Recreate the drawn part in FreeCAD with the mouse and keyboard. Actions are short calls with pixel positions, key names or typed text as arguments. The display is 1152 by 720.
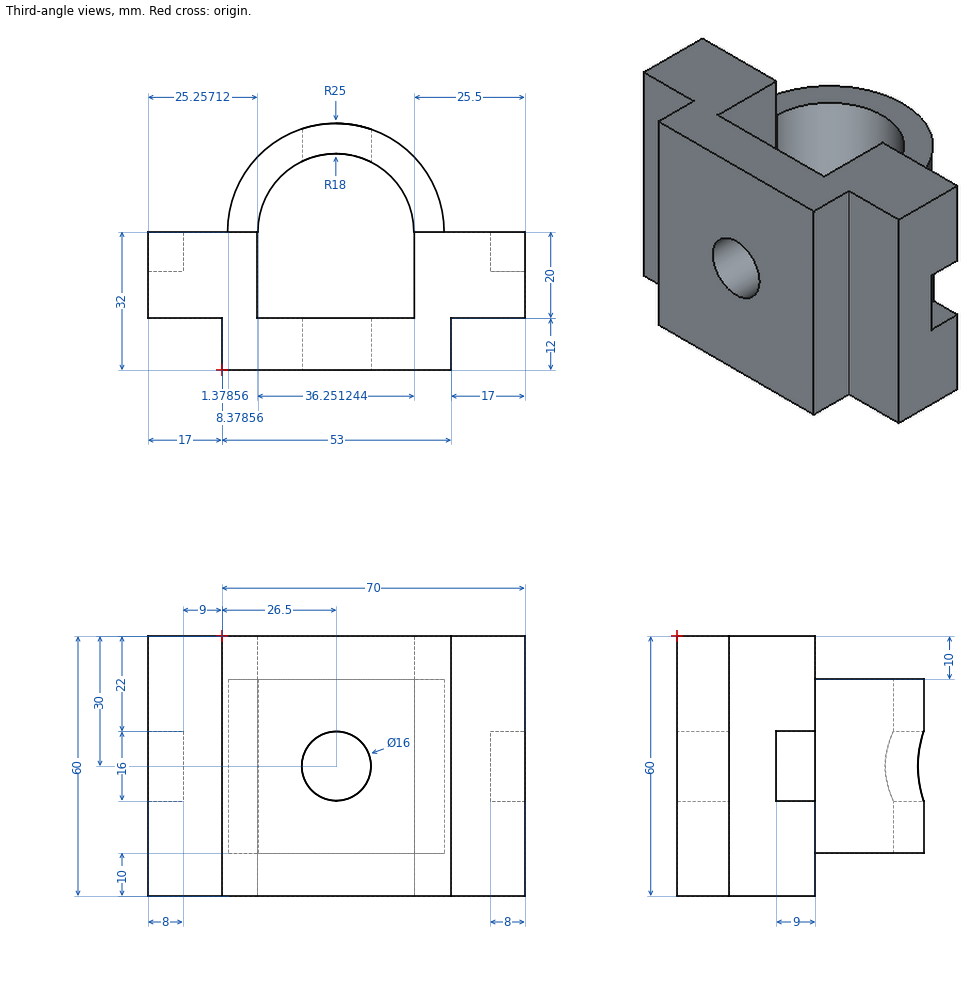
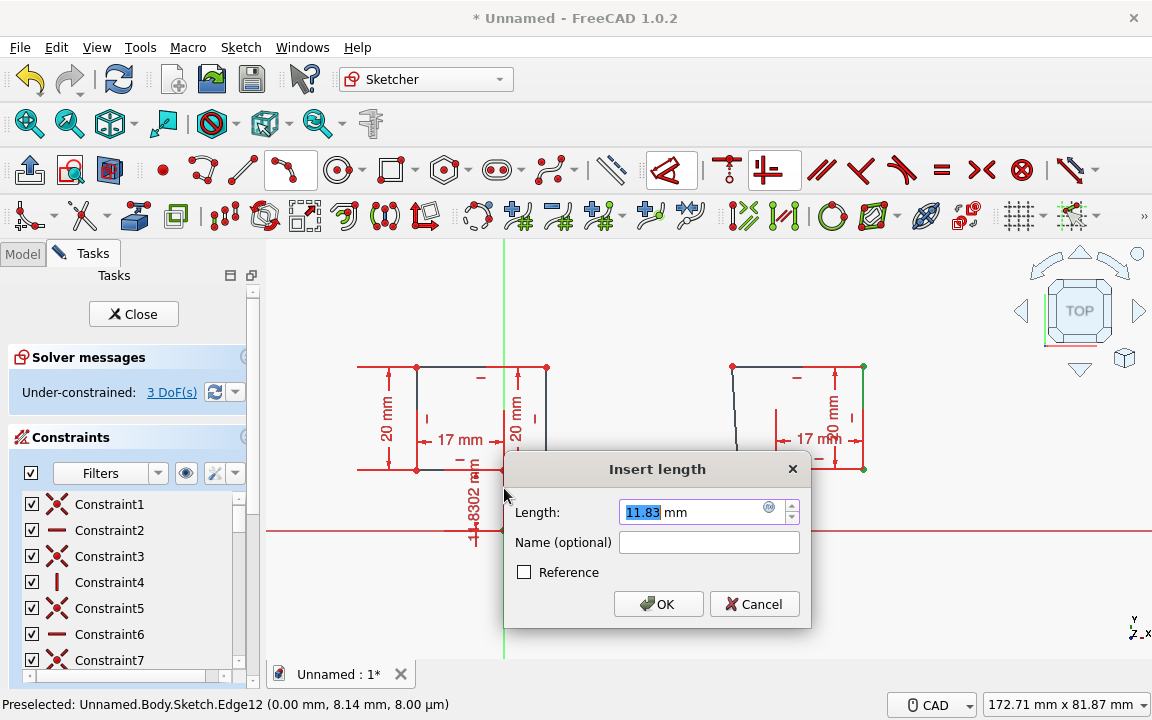
text(12)
key(Return)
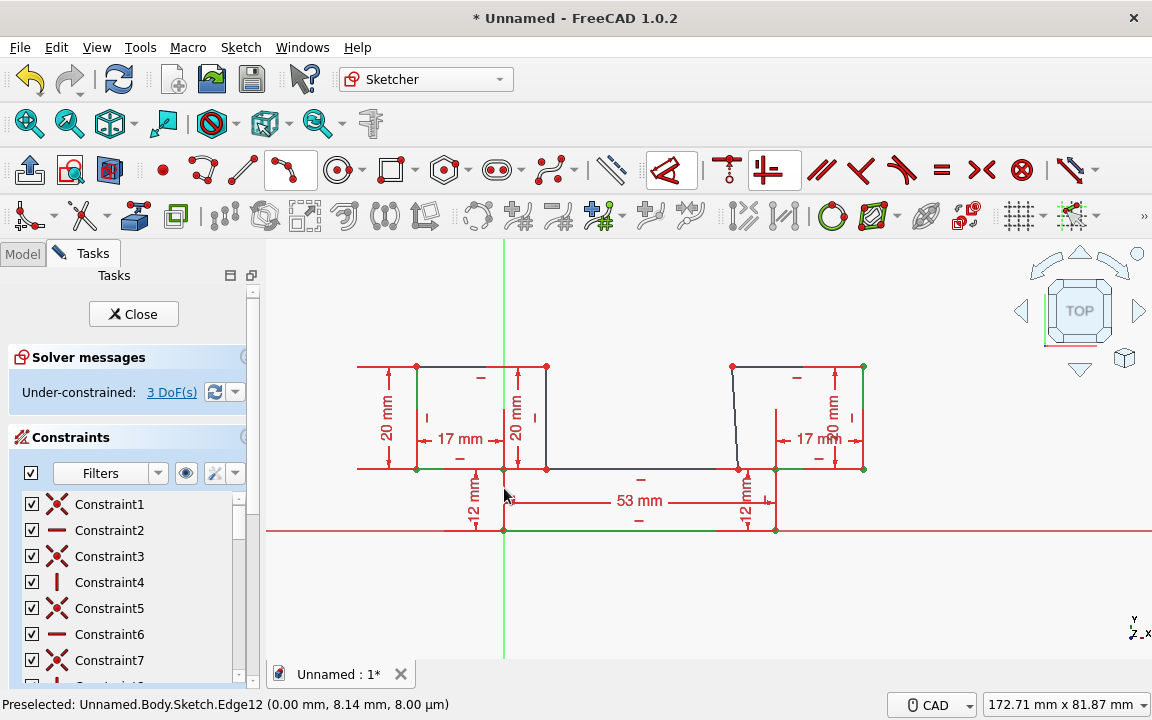
click(824, 367)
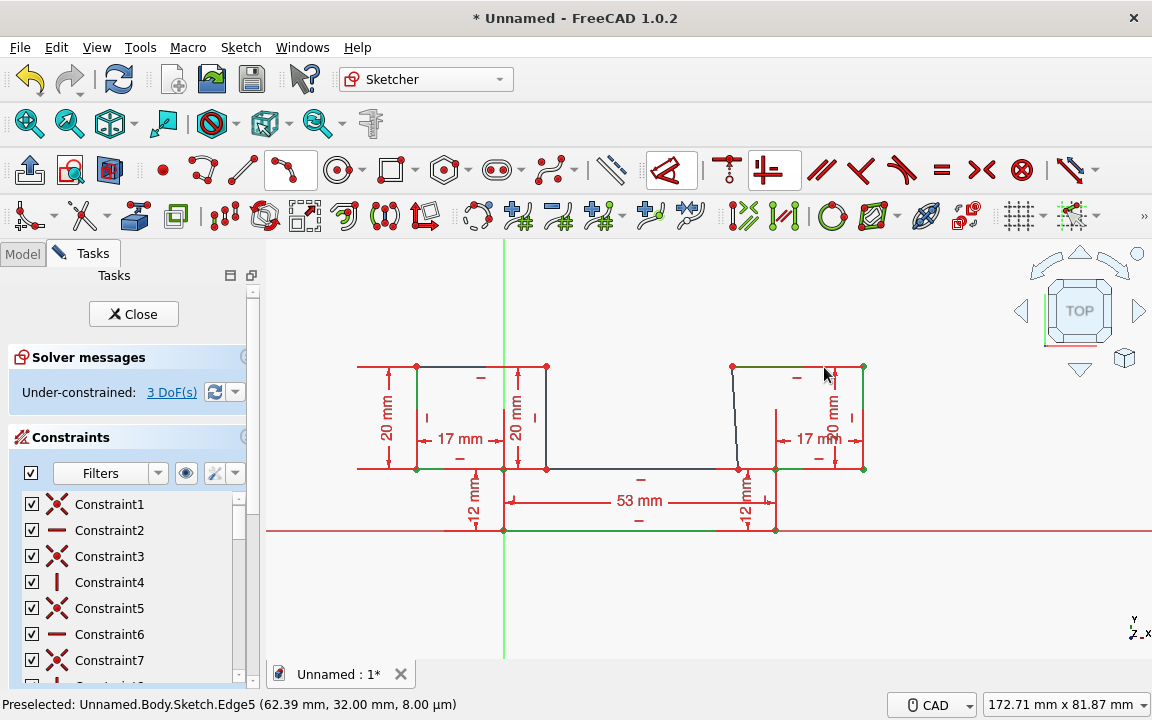
key(l)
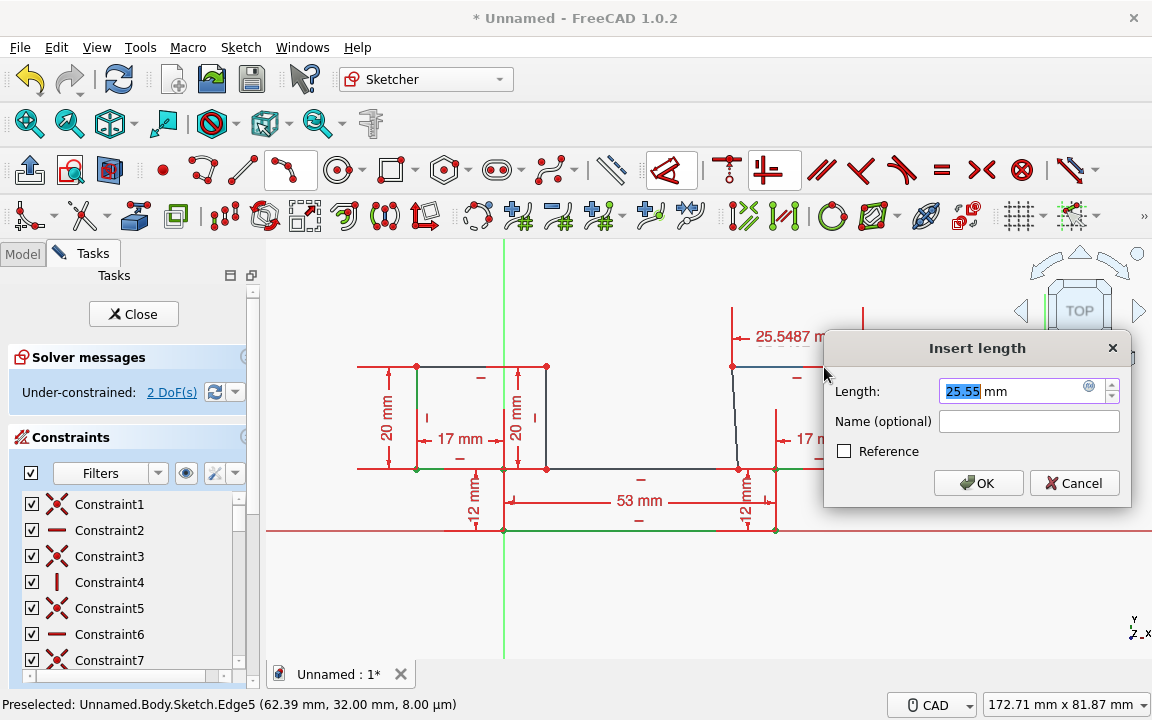
text(25.5)
key(Return)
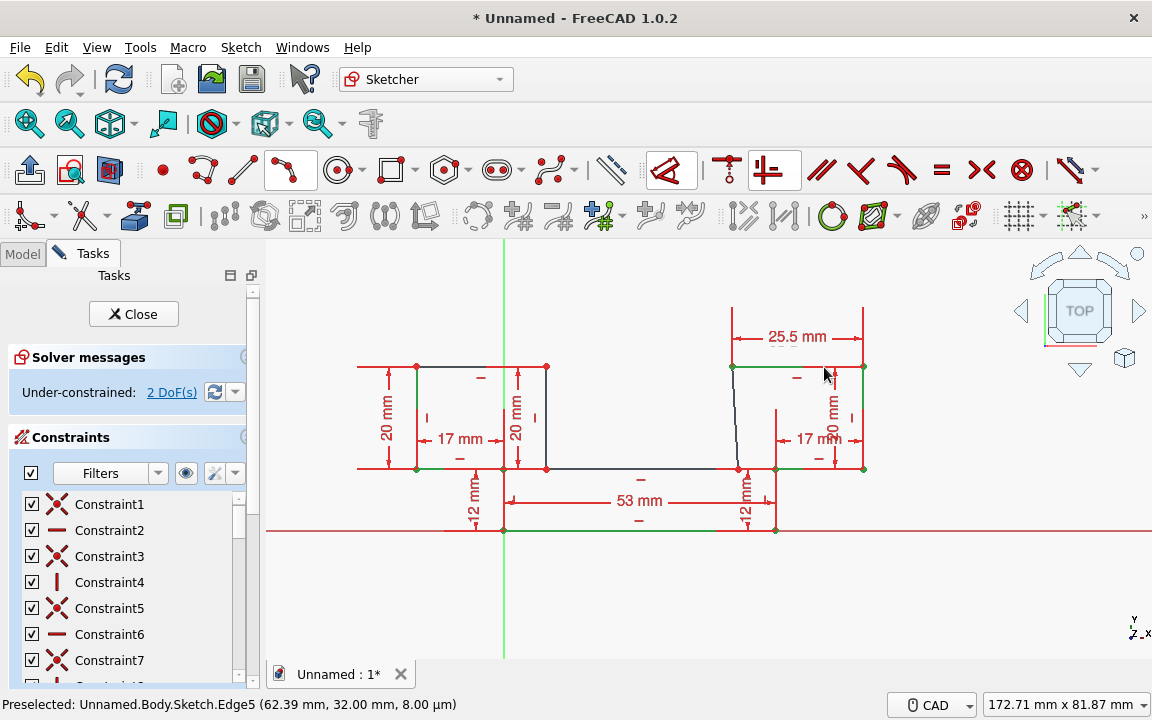
click(507, 367)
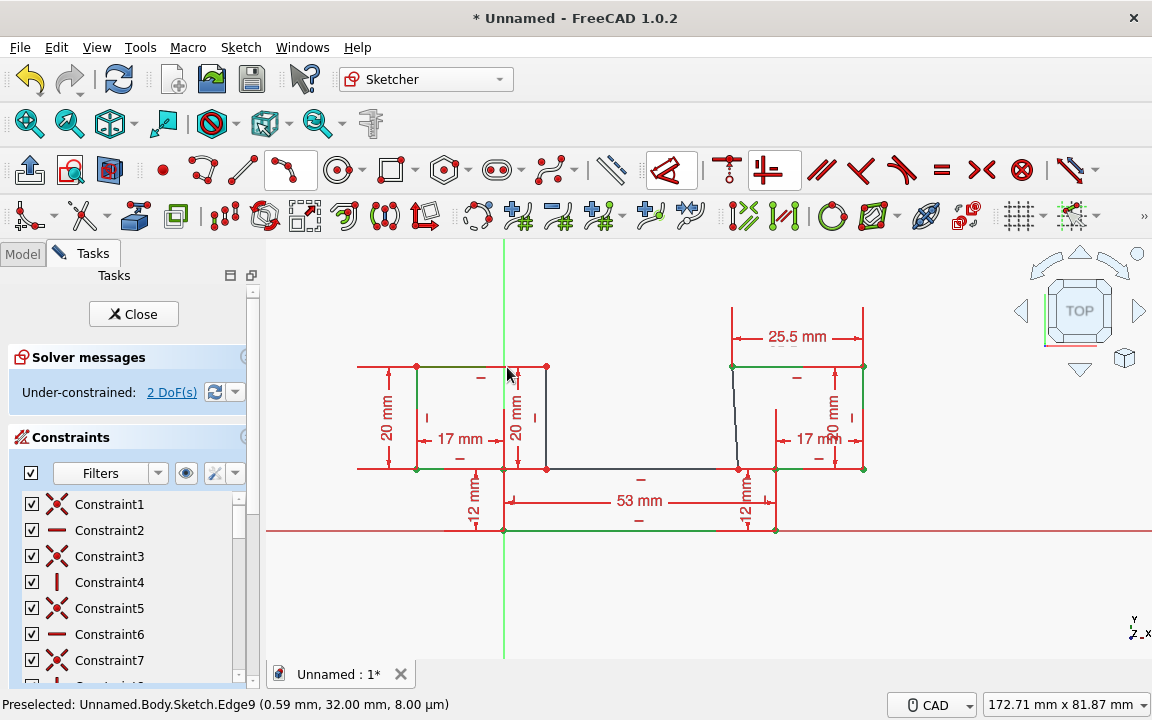
key(l)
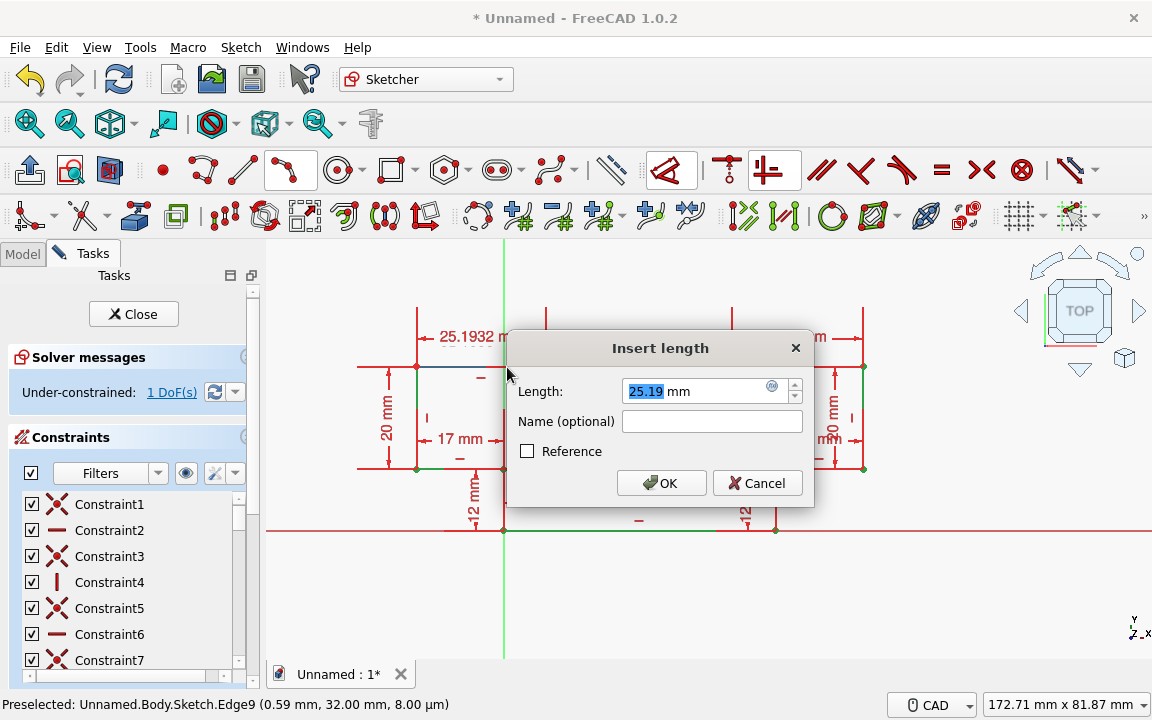
text(25.25712)
key(Return)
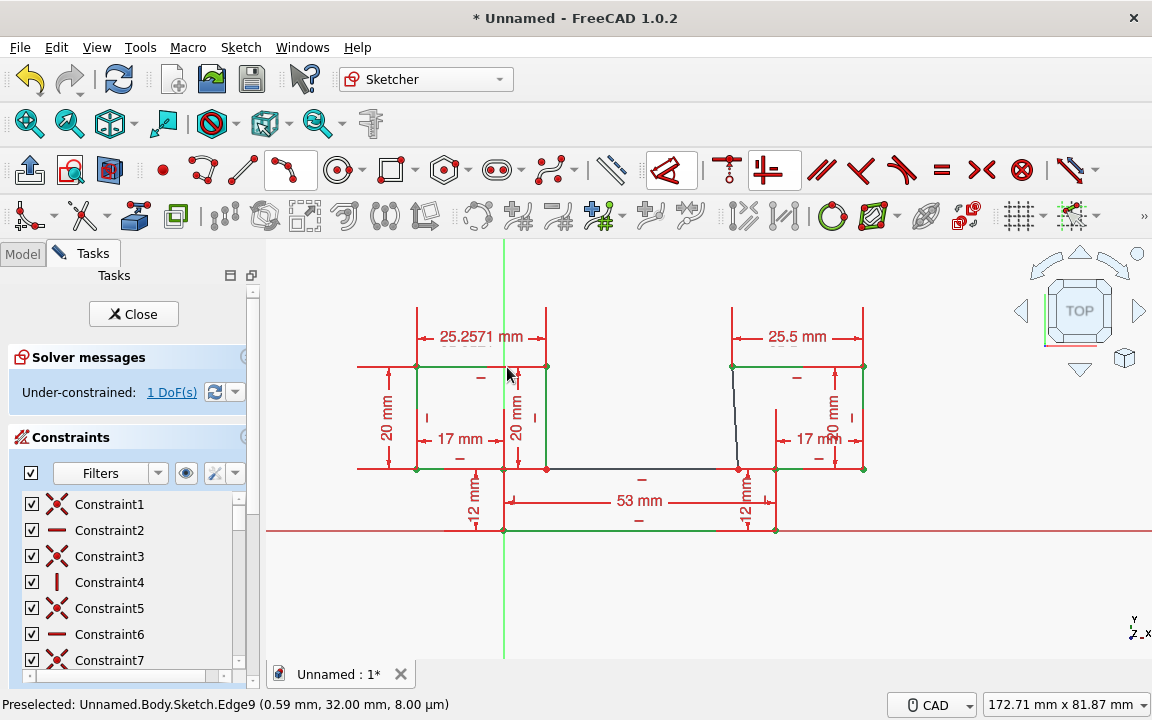
click(680, 469)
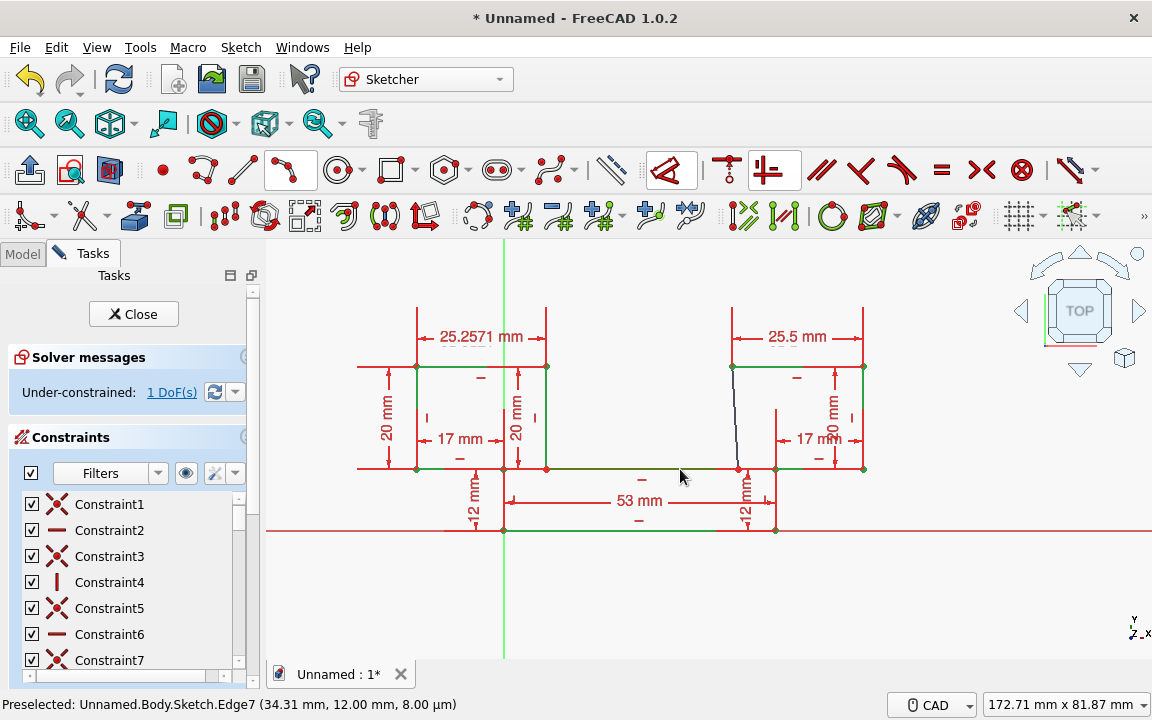
key(l)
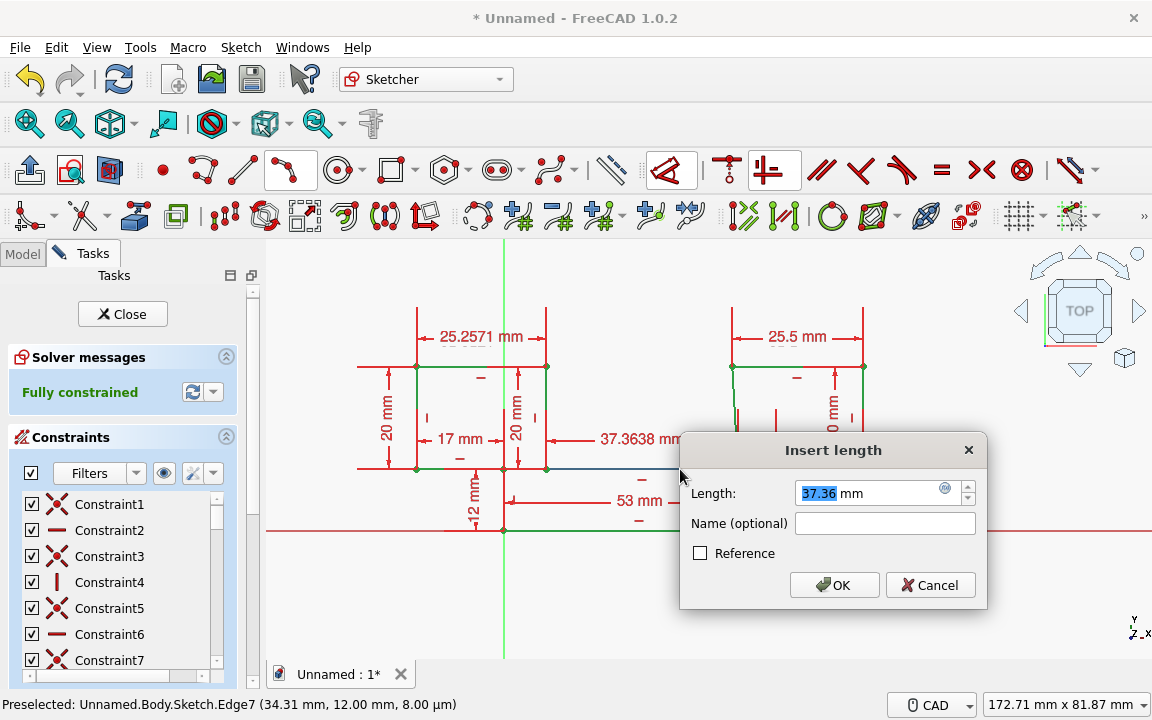
text(36.251244)
key(Return)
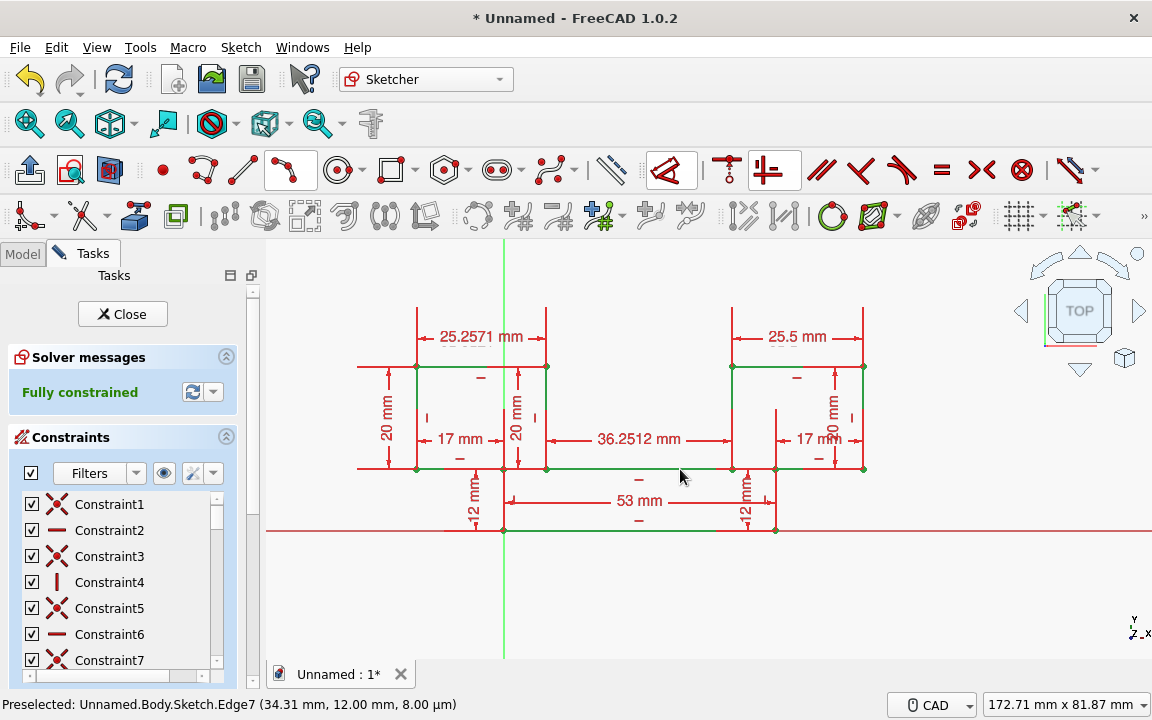
click(123, 314)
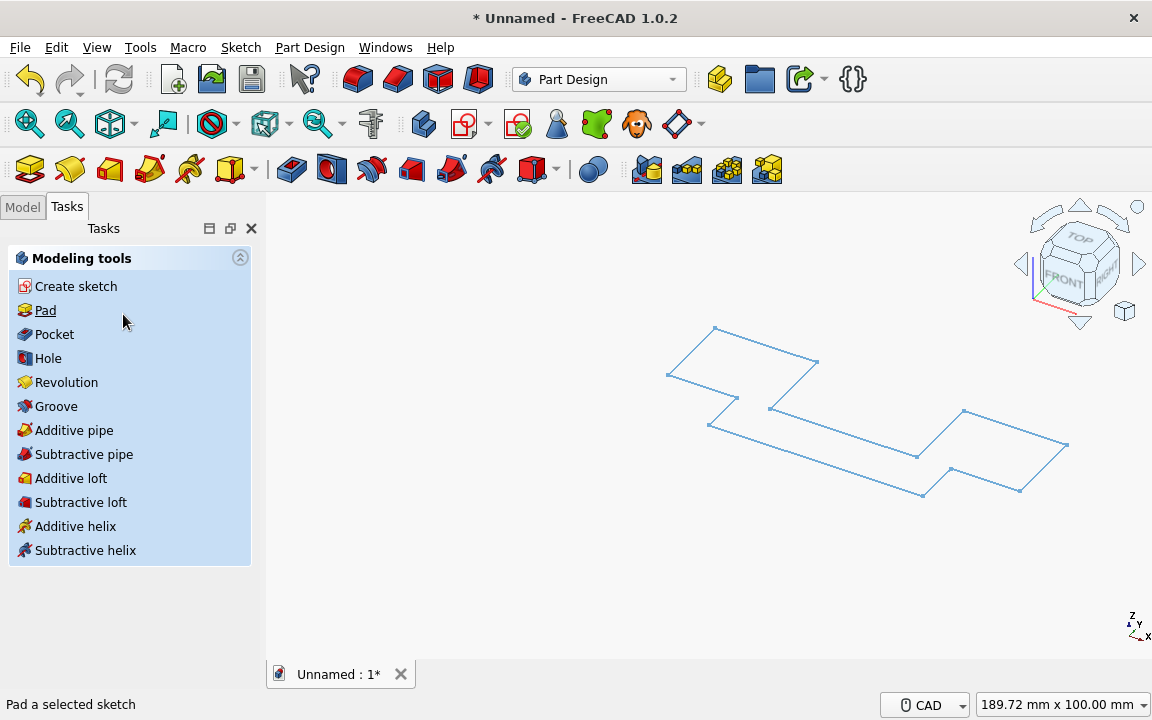
click(30, 170)